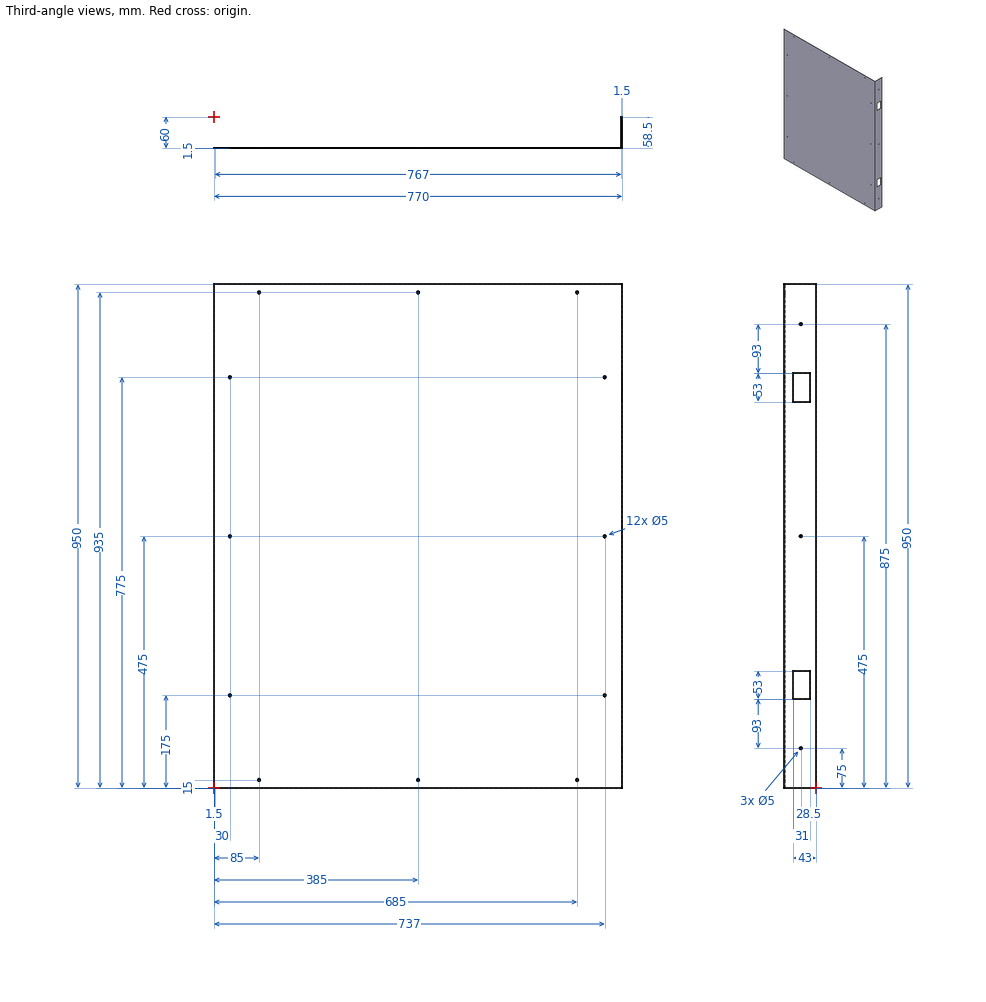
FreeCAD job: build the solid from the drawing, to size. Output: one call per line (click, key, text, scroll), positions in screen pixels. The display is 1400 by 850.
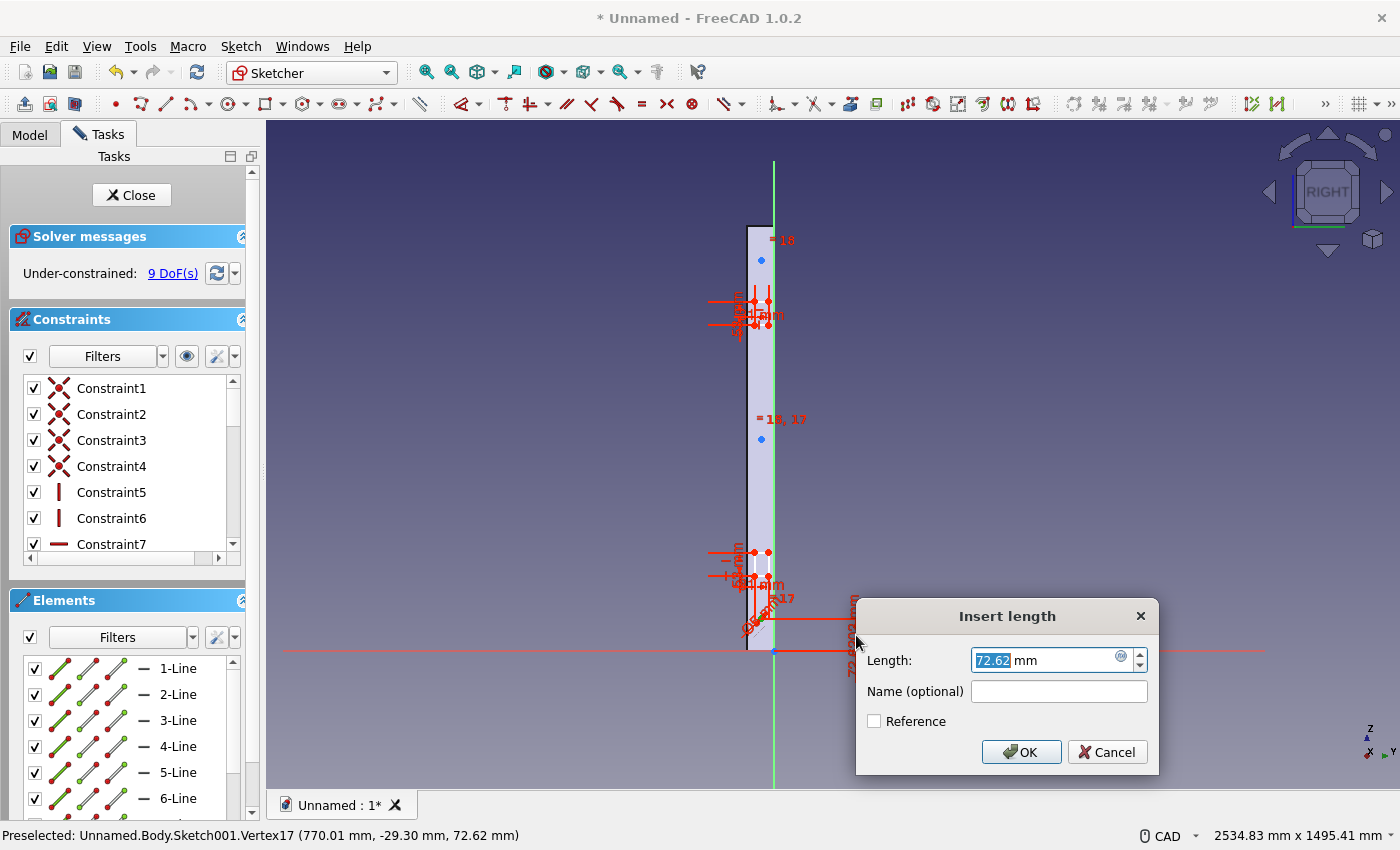
text(75)
key(Return)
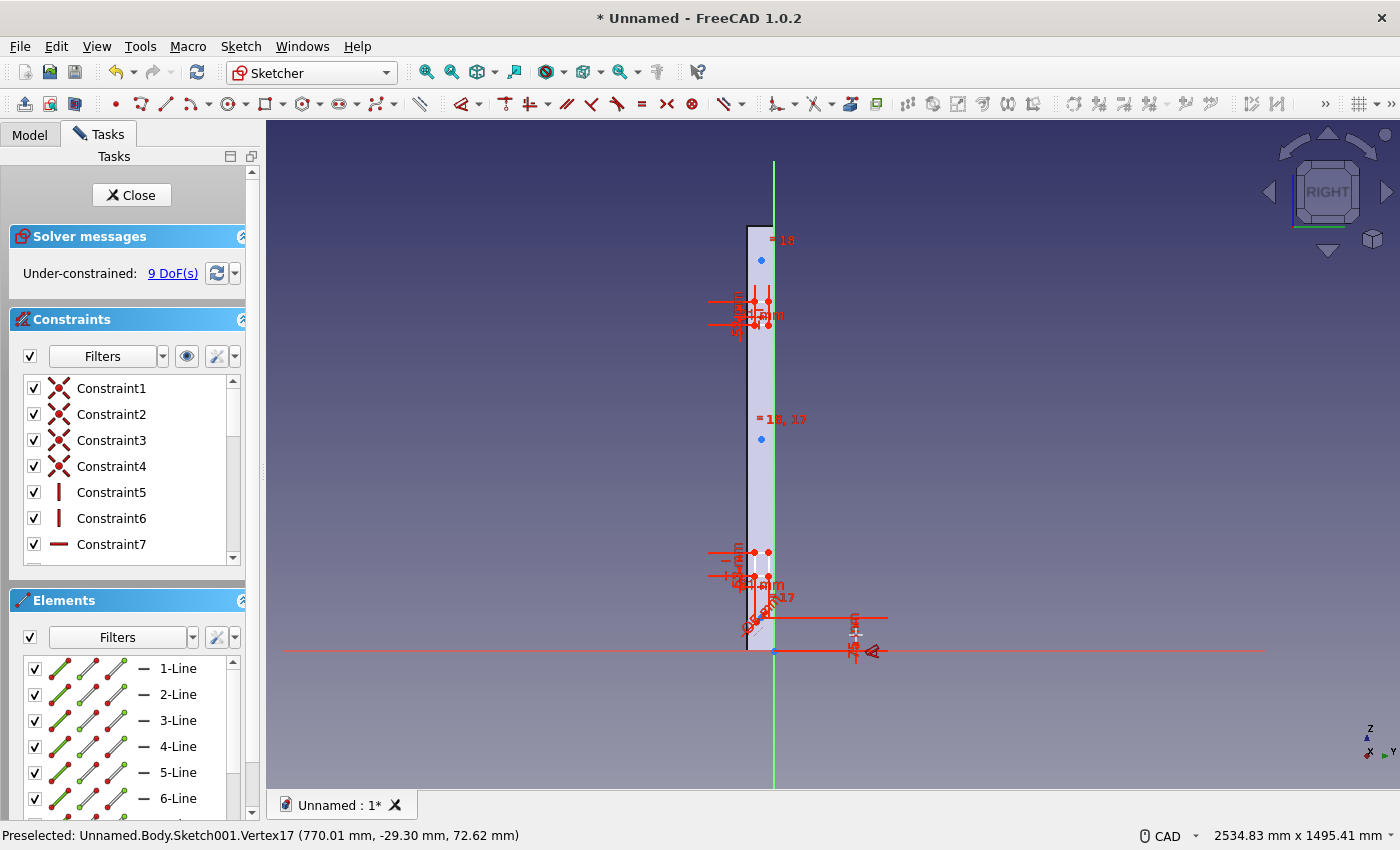
scroll(755, 553, up, 4)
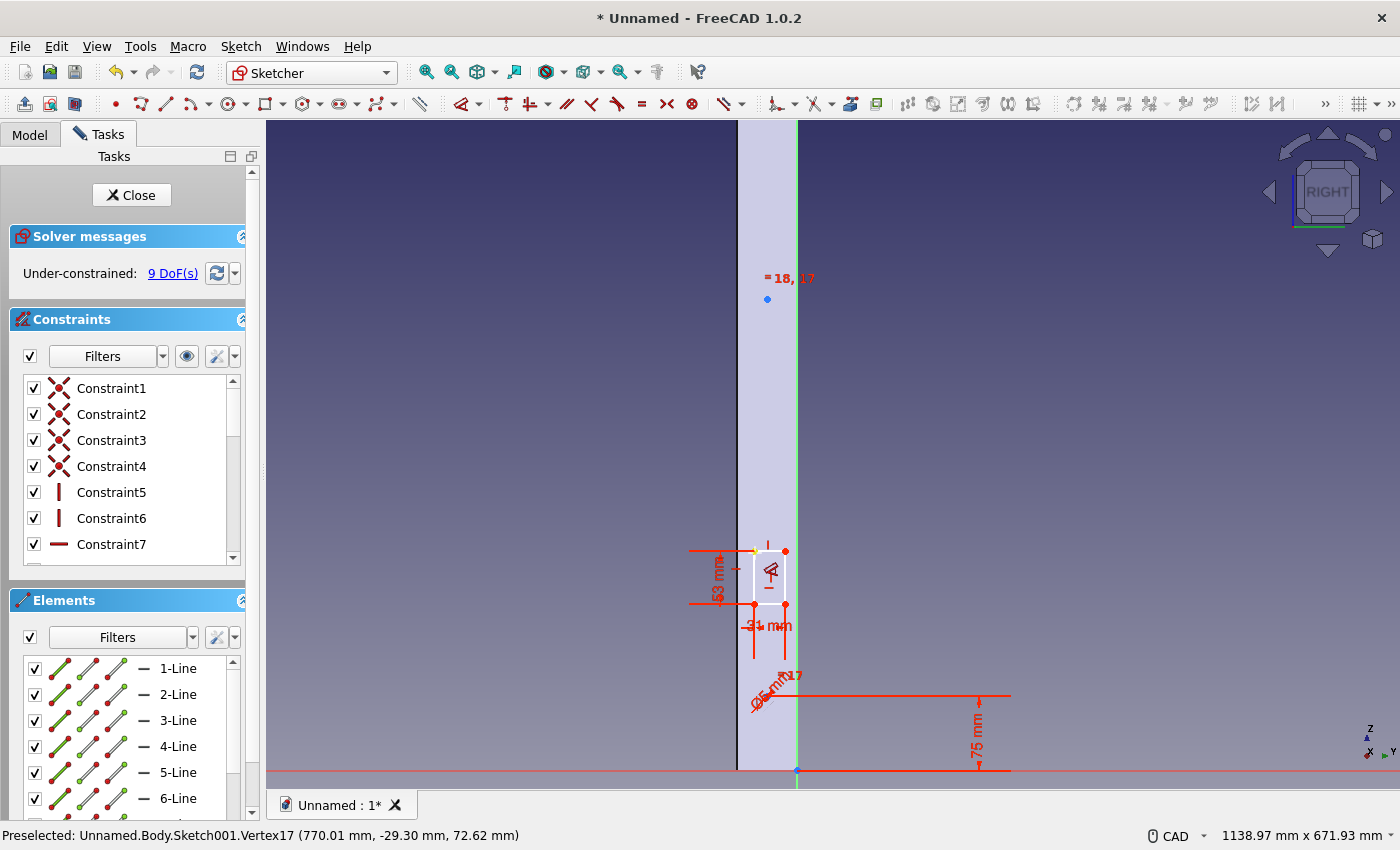
click(754, 551)
click(776, 517)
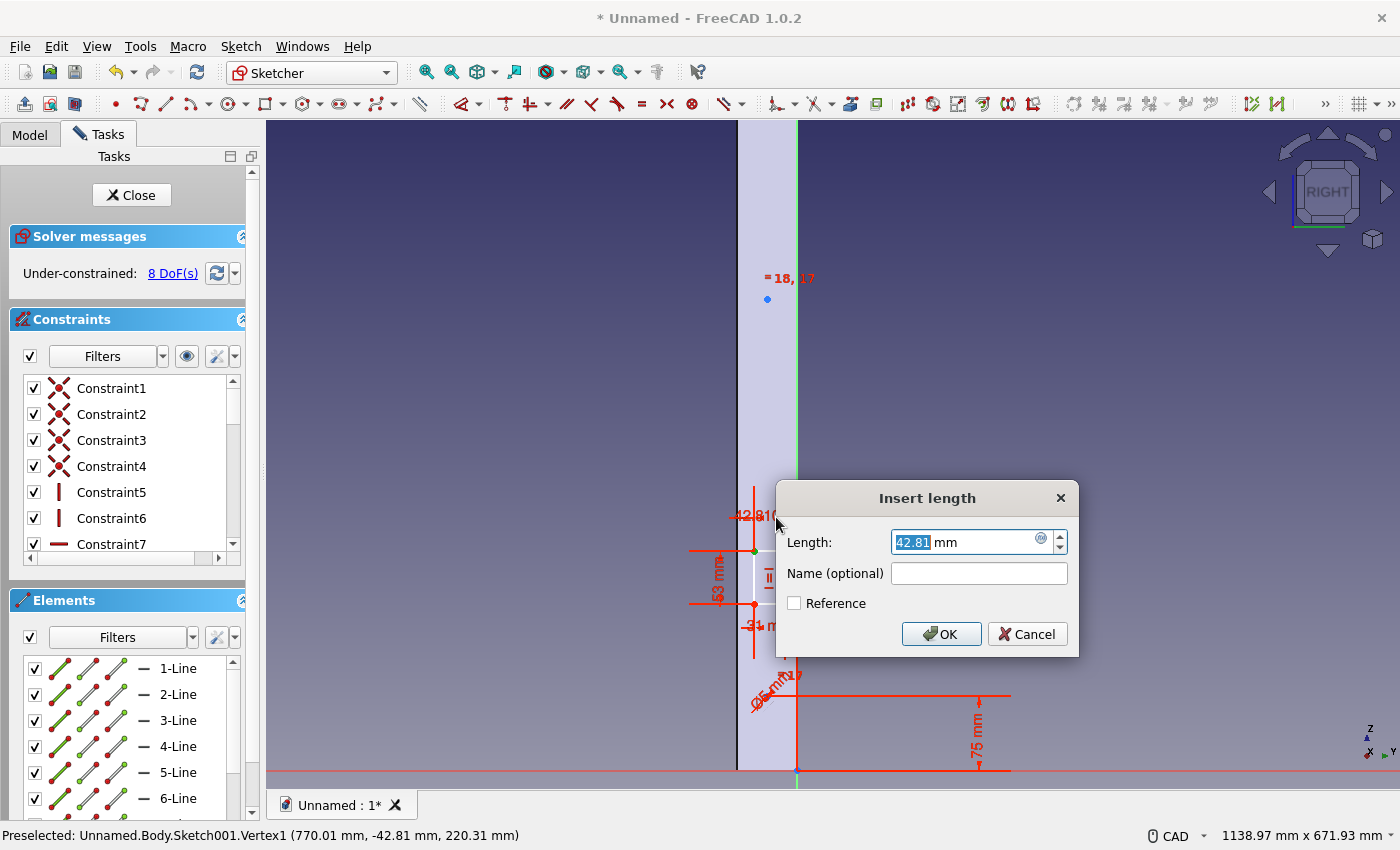
text(43)
key(Return)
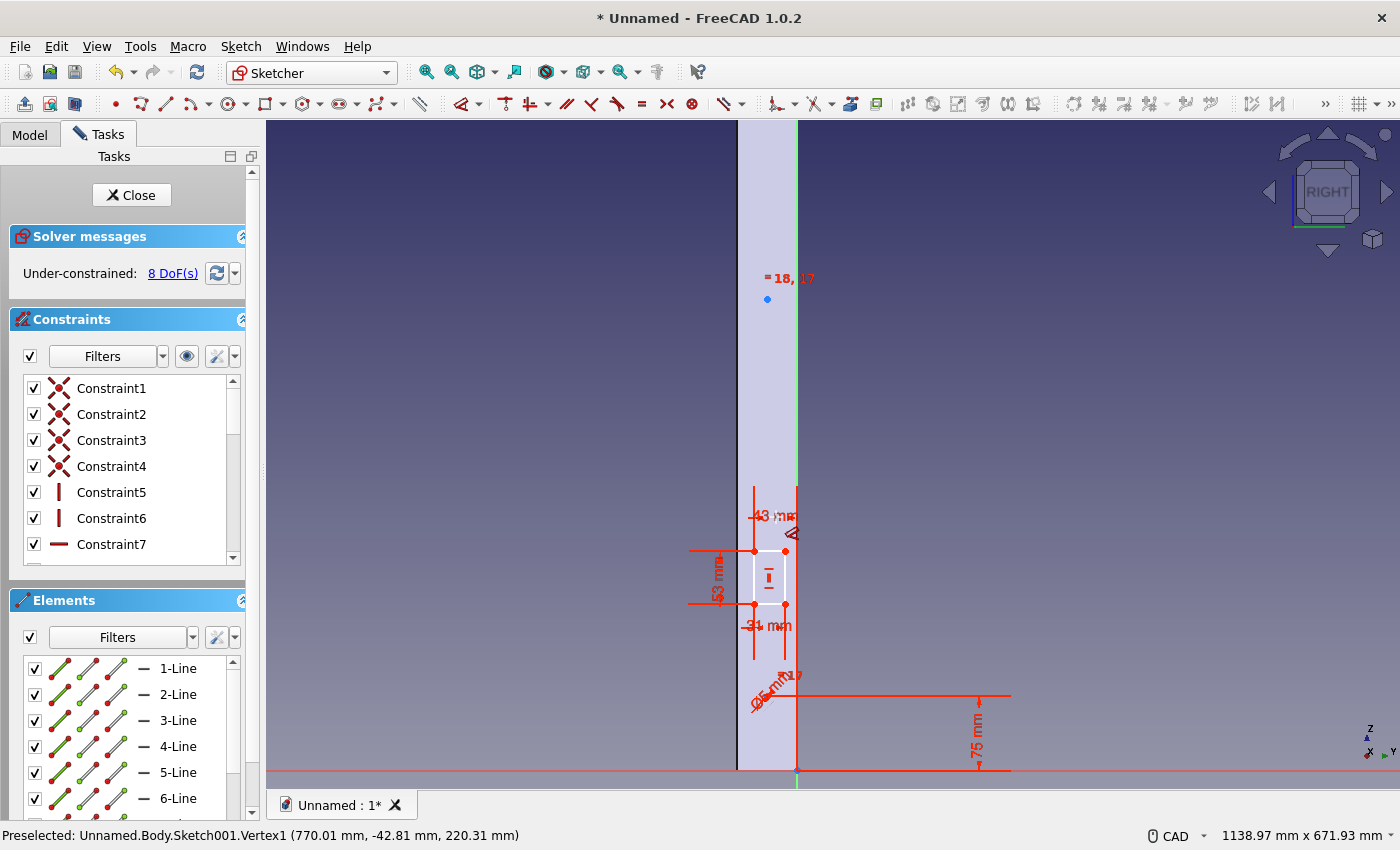
scroll(755, 553, down, 4)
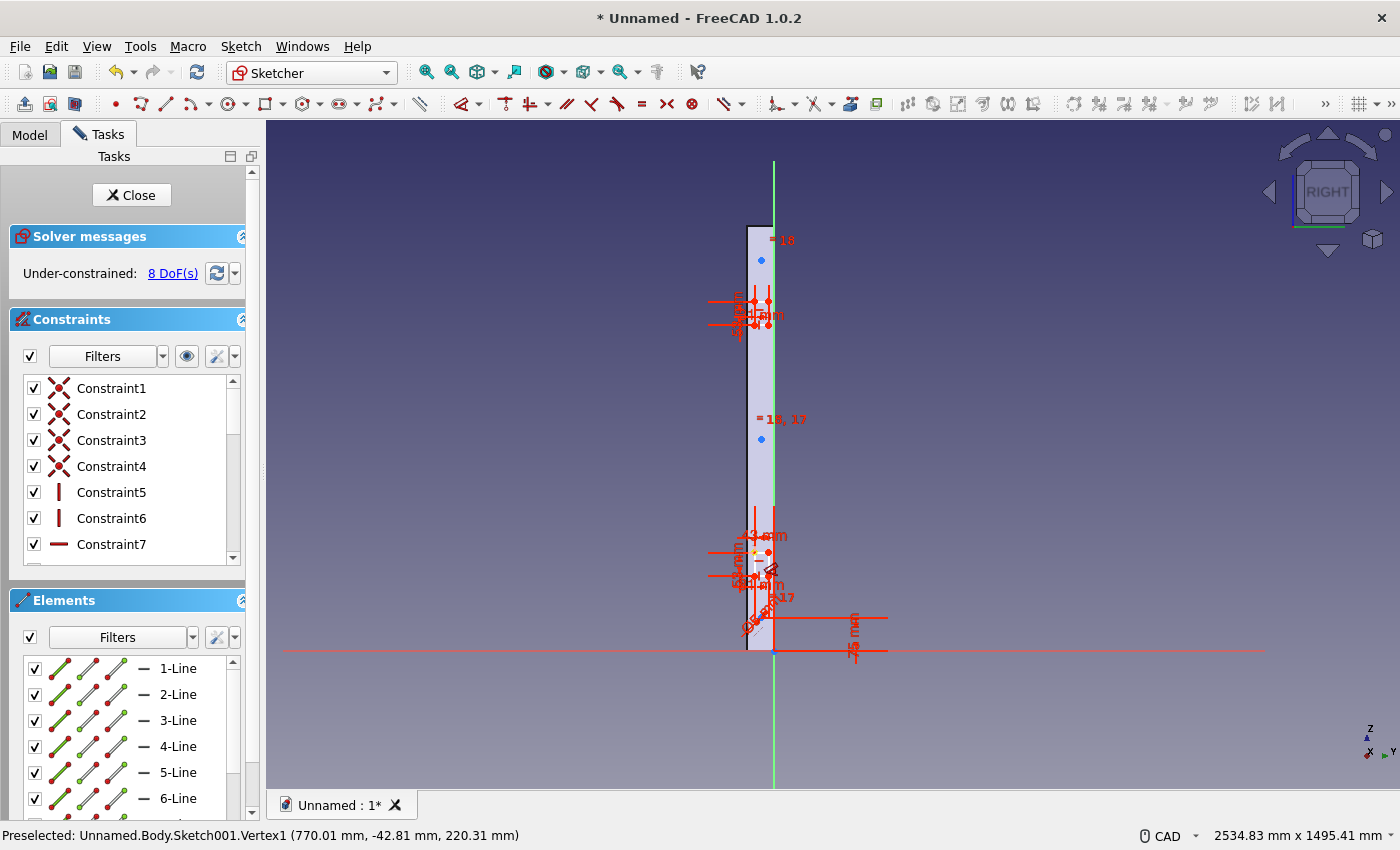
scroll(755, 302, up, 4)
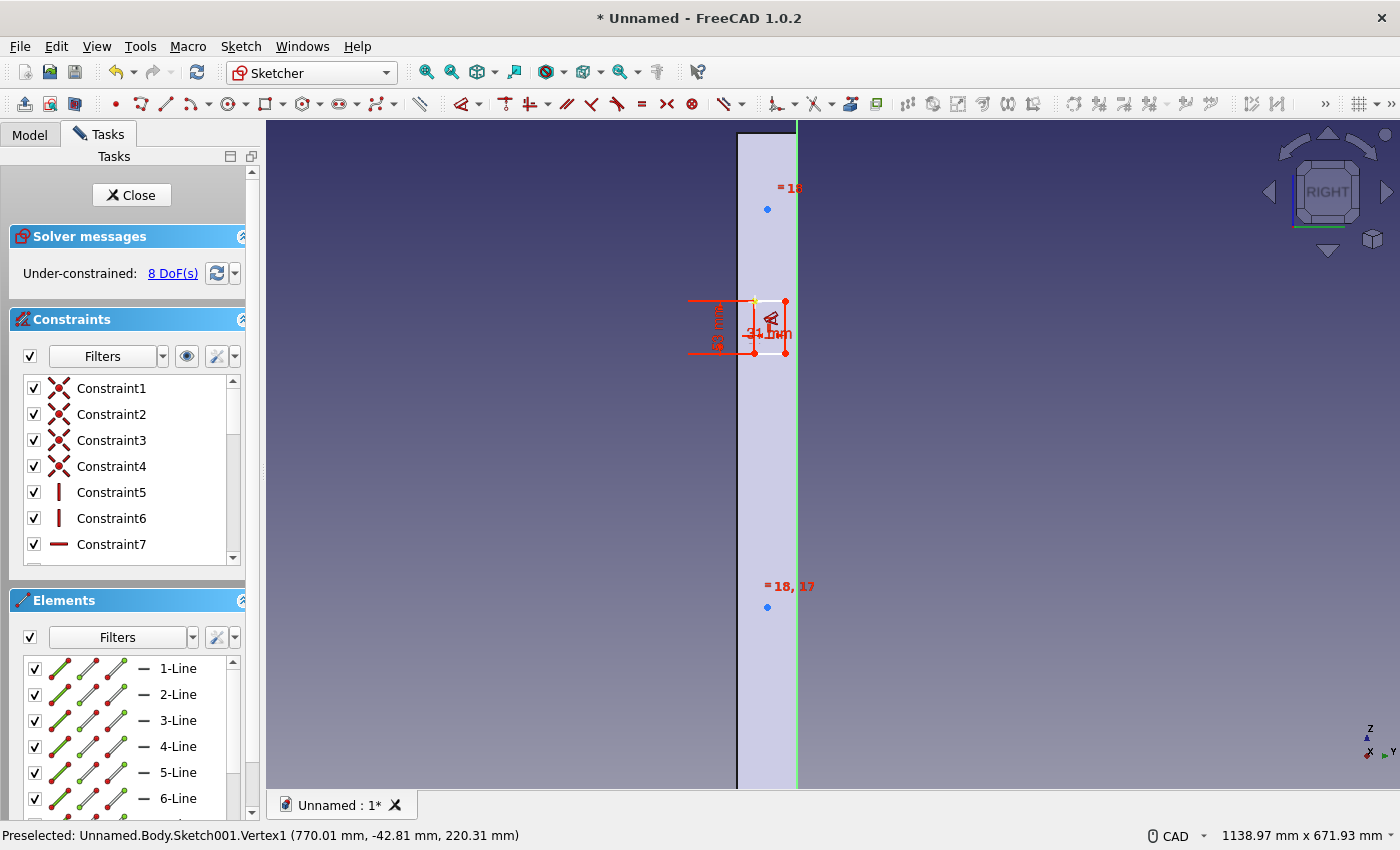
click(754, 301)
click(776, 267)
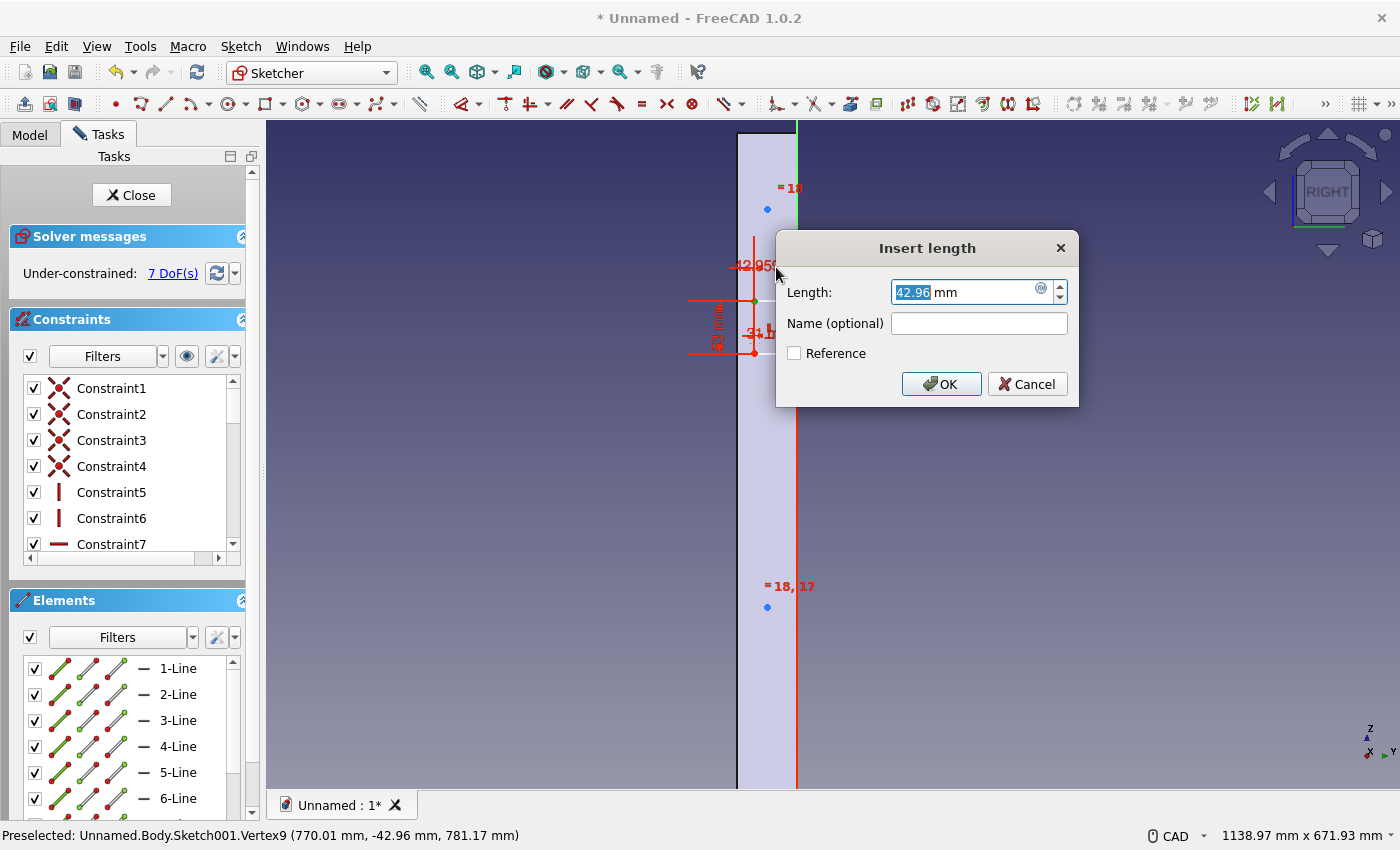
text(43)
key(Return)